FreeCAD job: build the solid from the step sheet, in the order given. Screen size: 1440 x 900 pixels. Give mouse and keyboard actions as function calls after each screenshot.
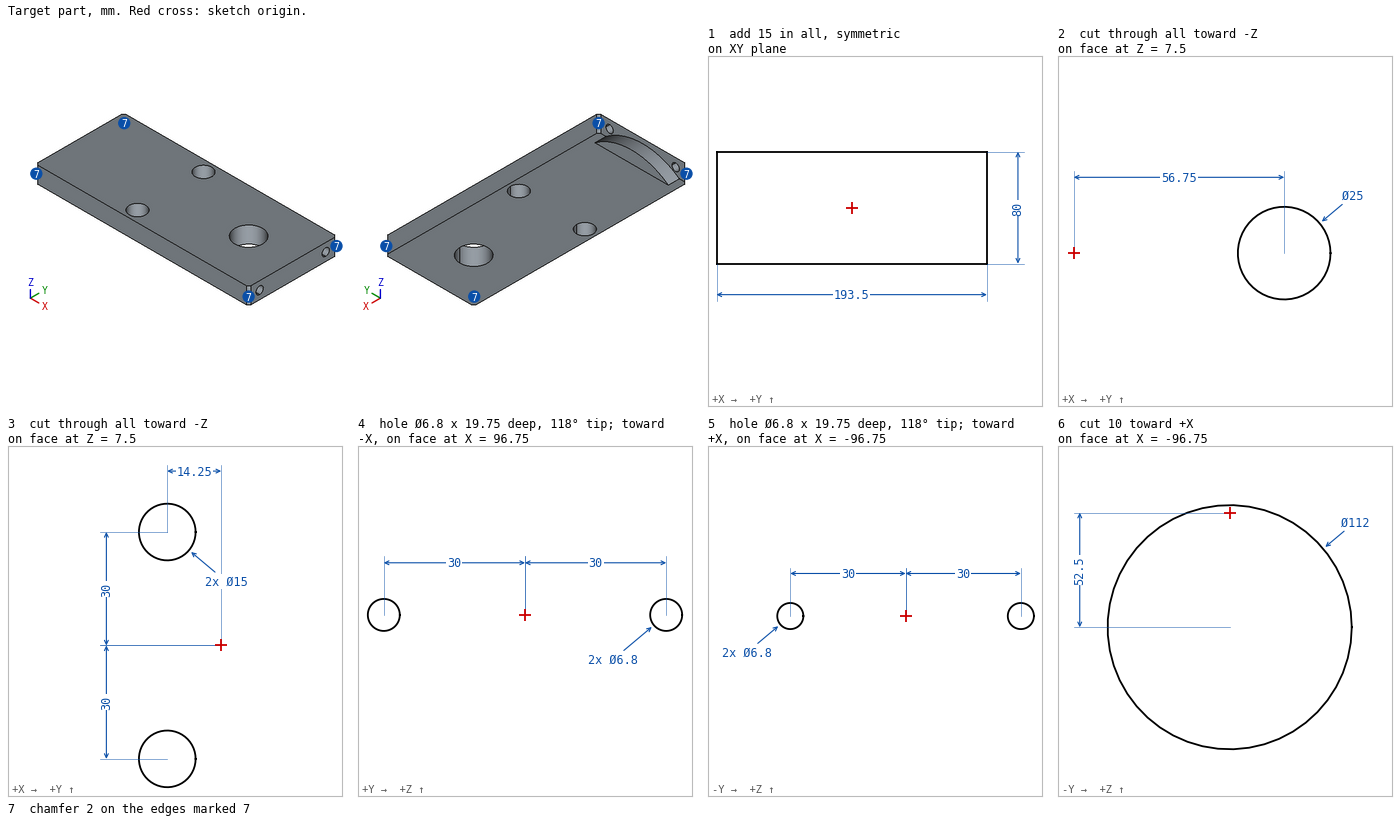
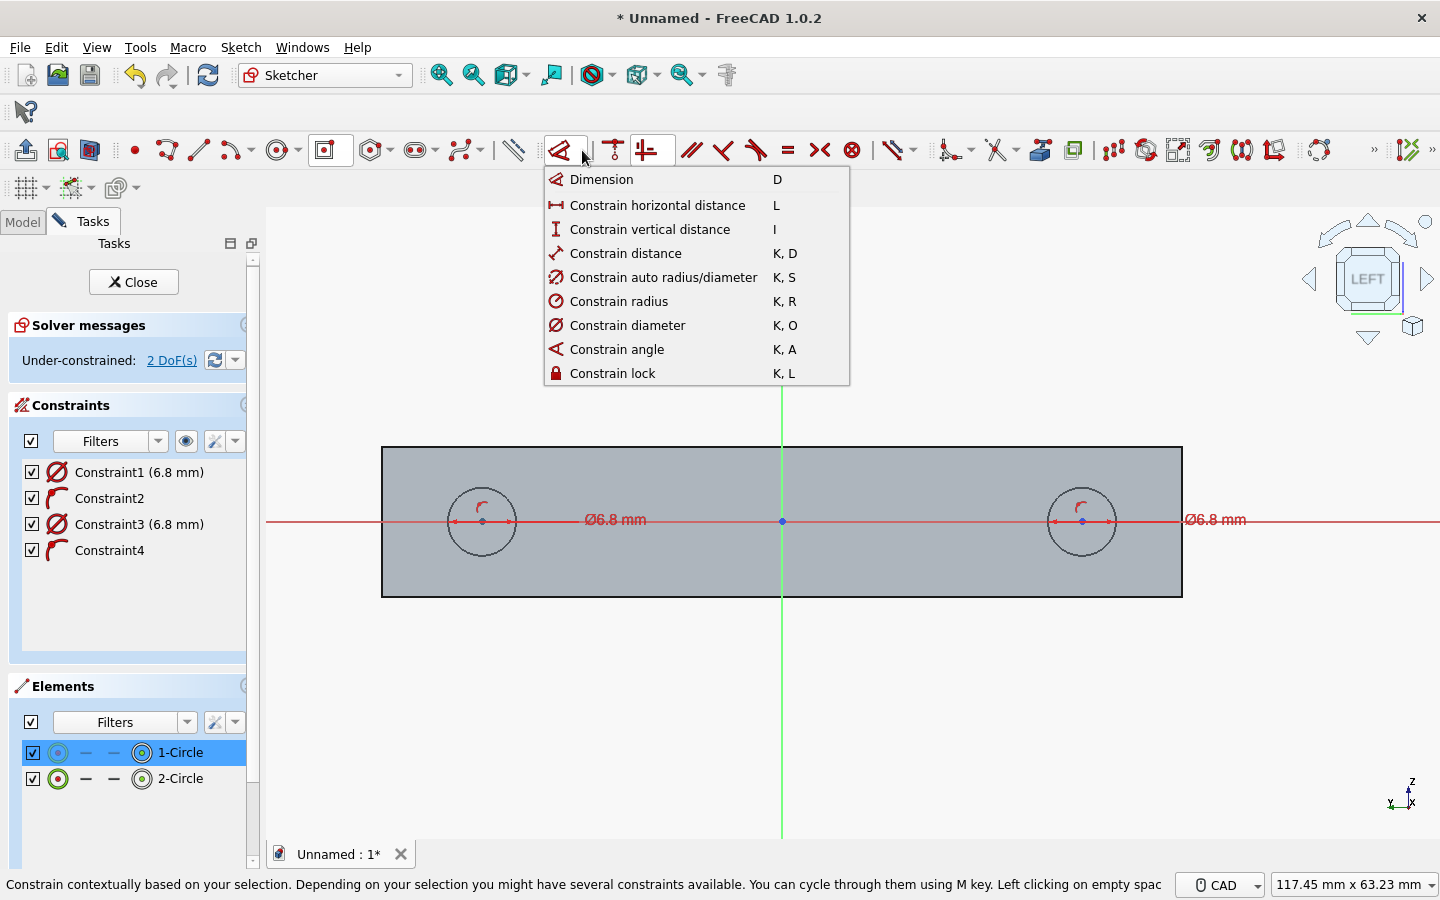
click(697, 205)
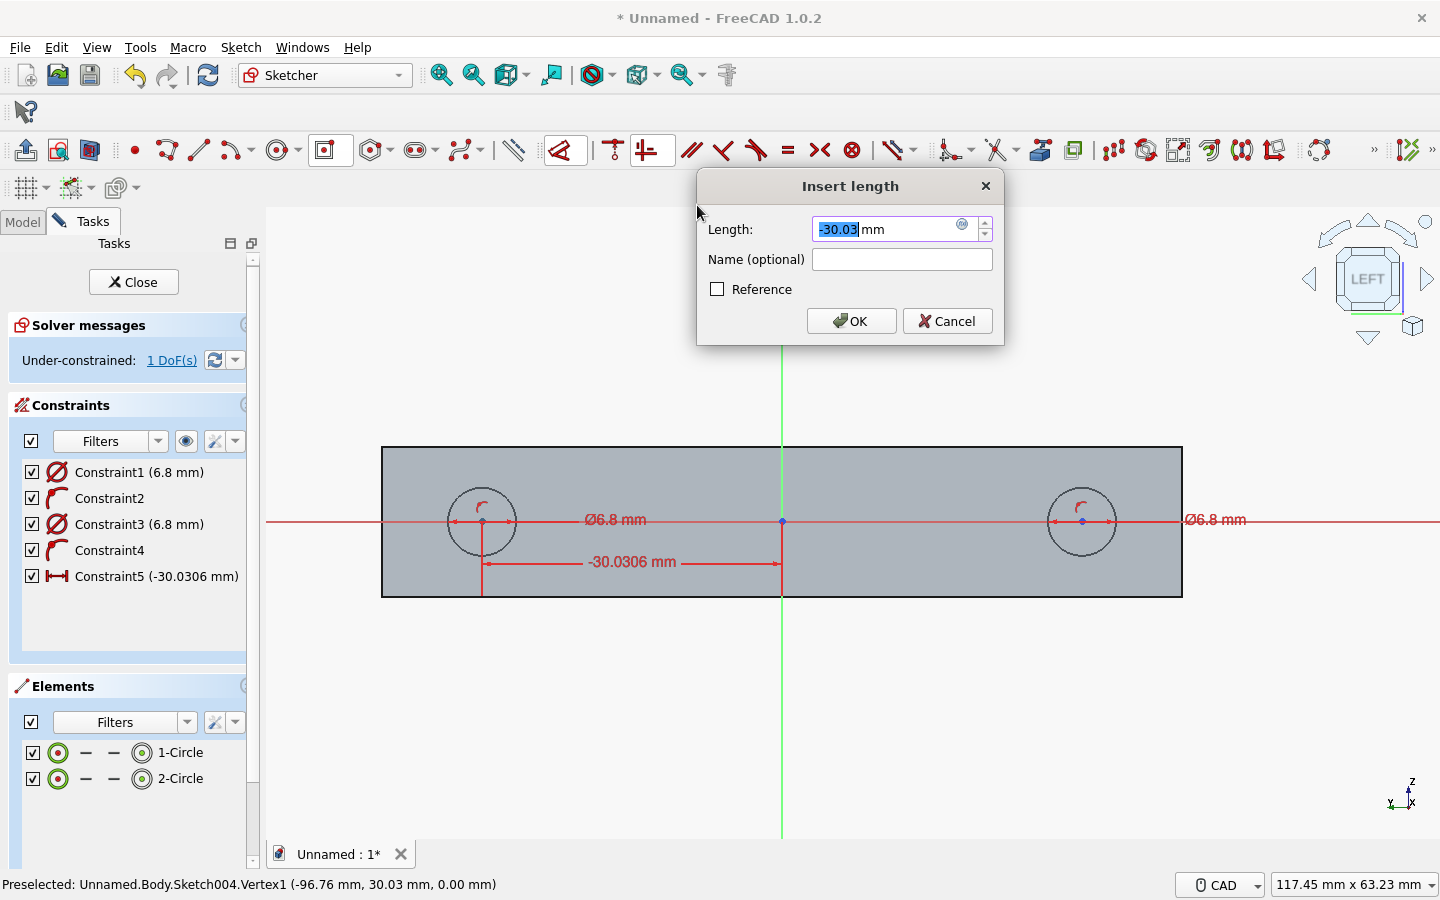
text(-30)
key(Return)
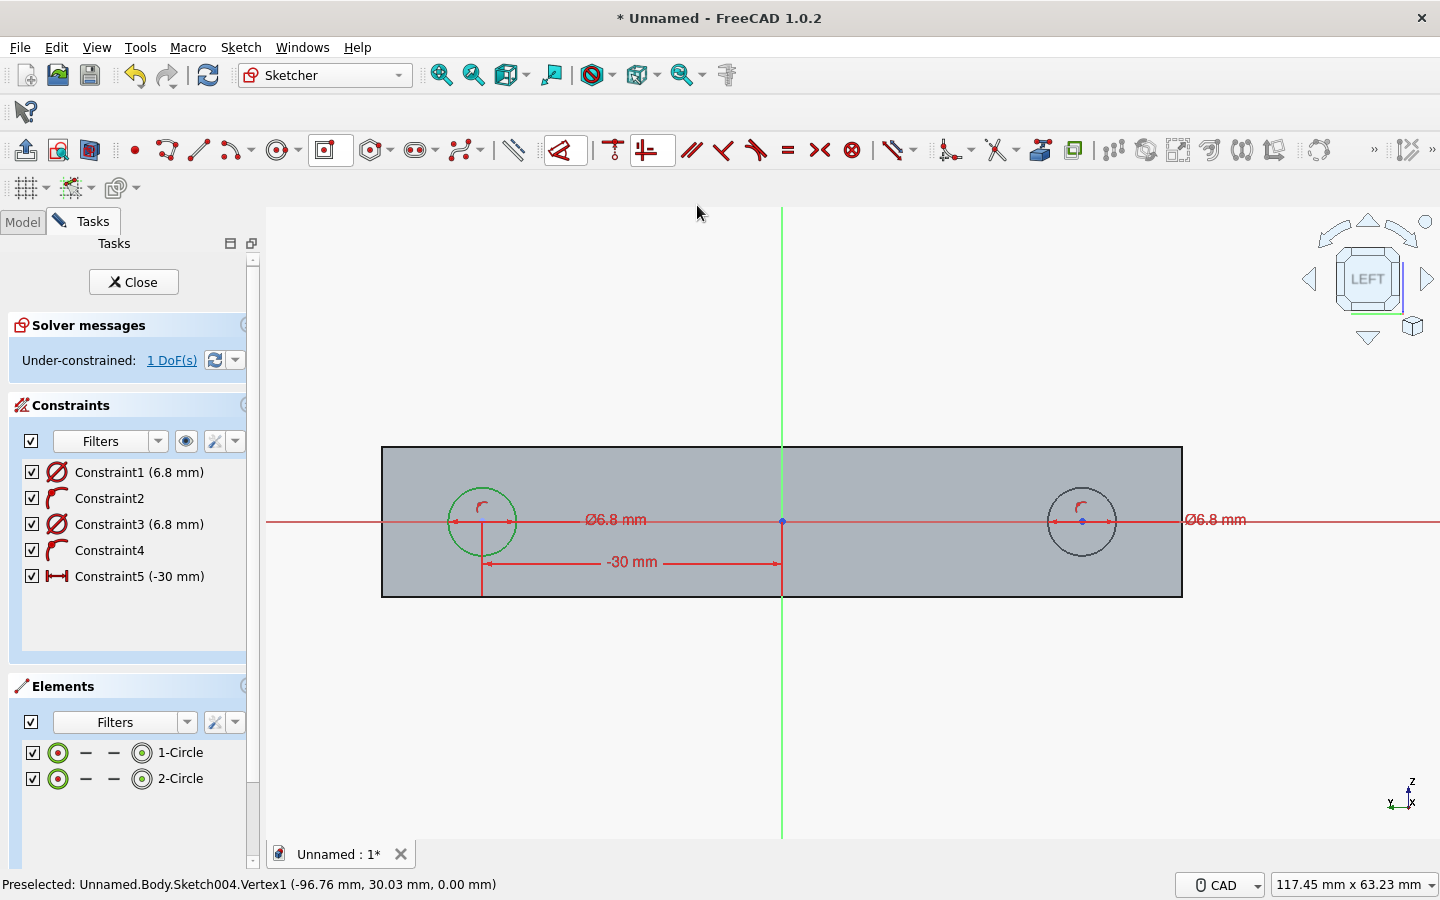
click(1082, 522)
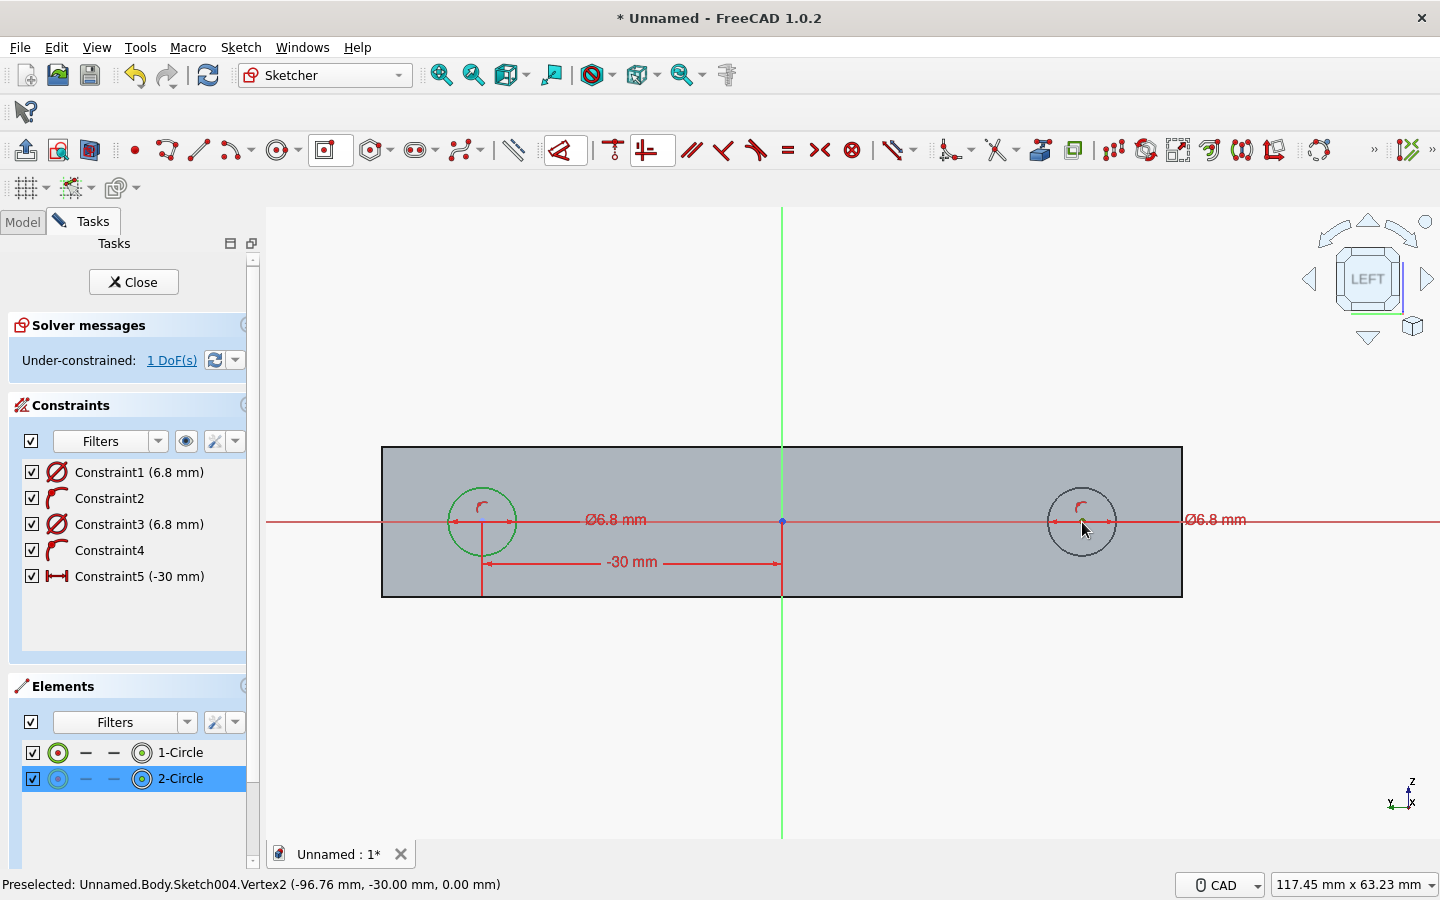
click(582, 150)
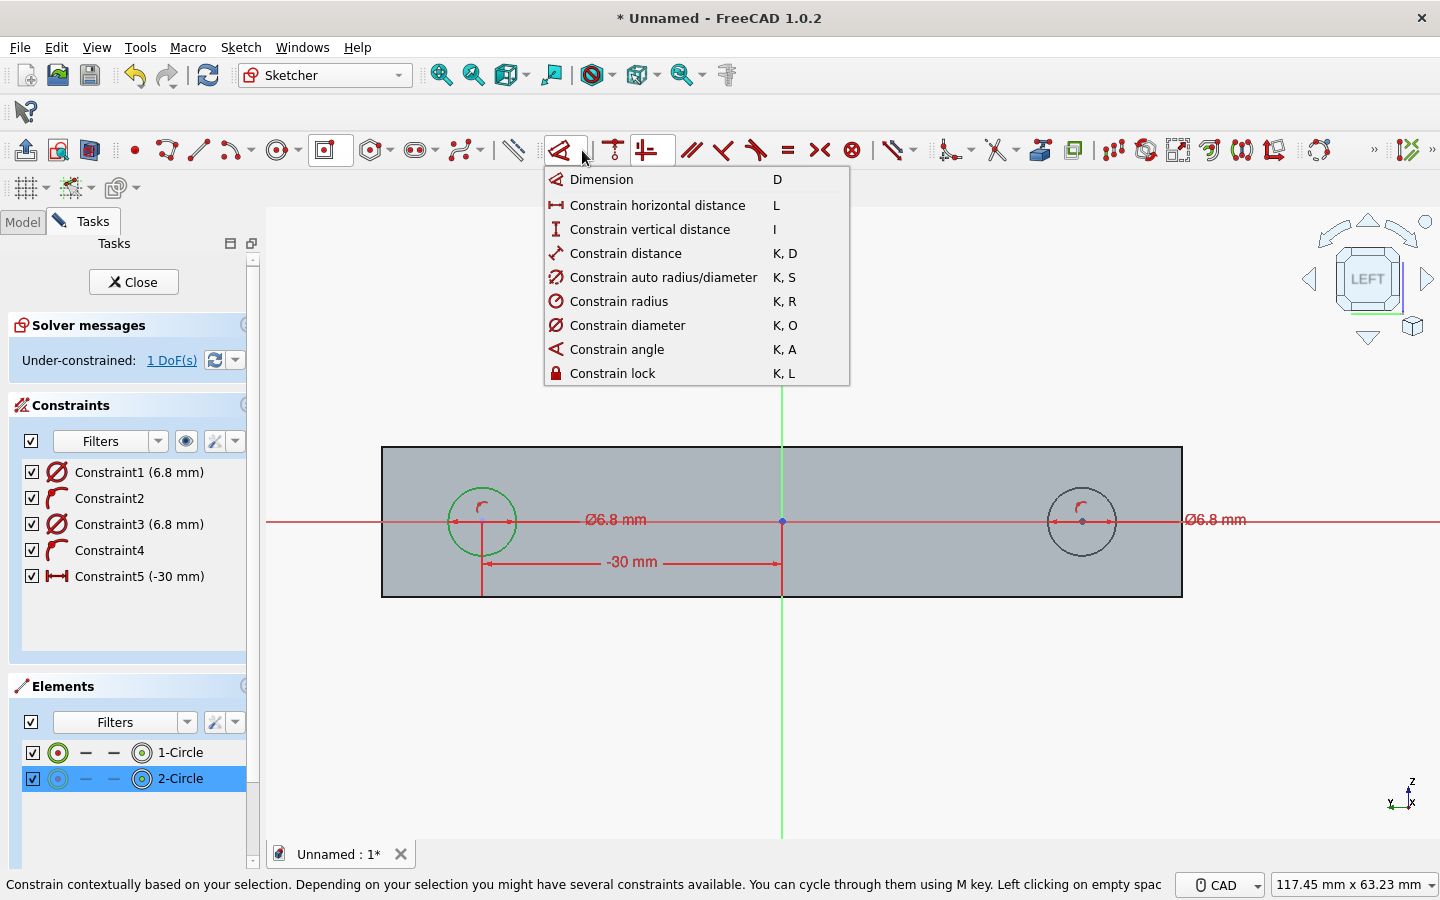
click(697, 205)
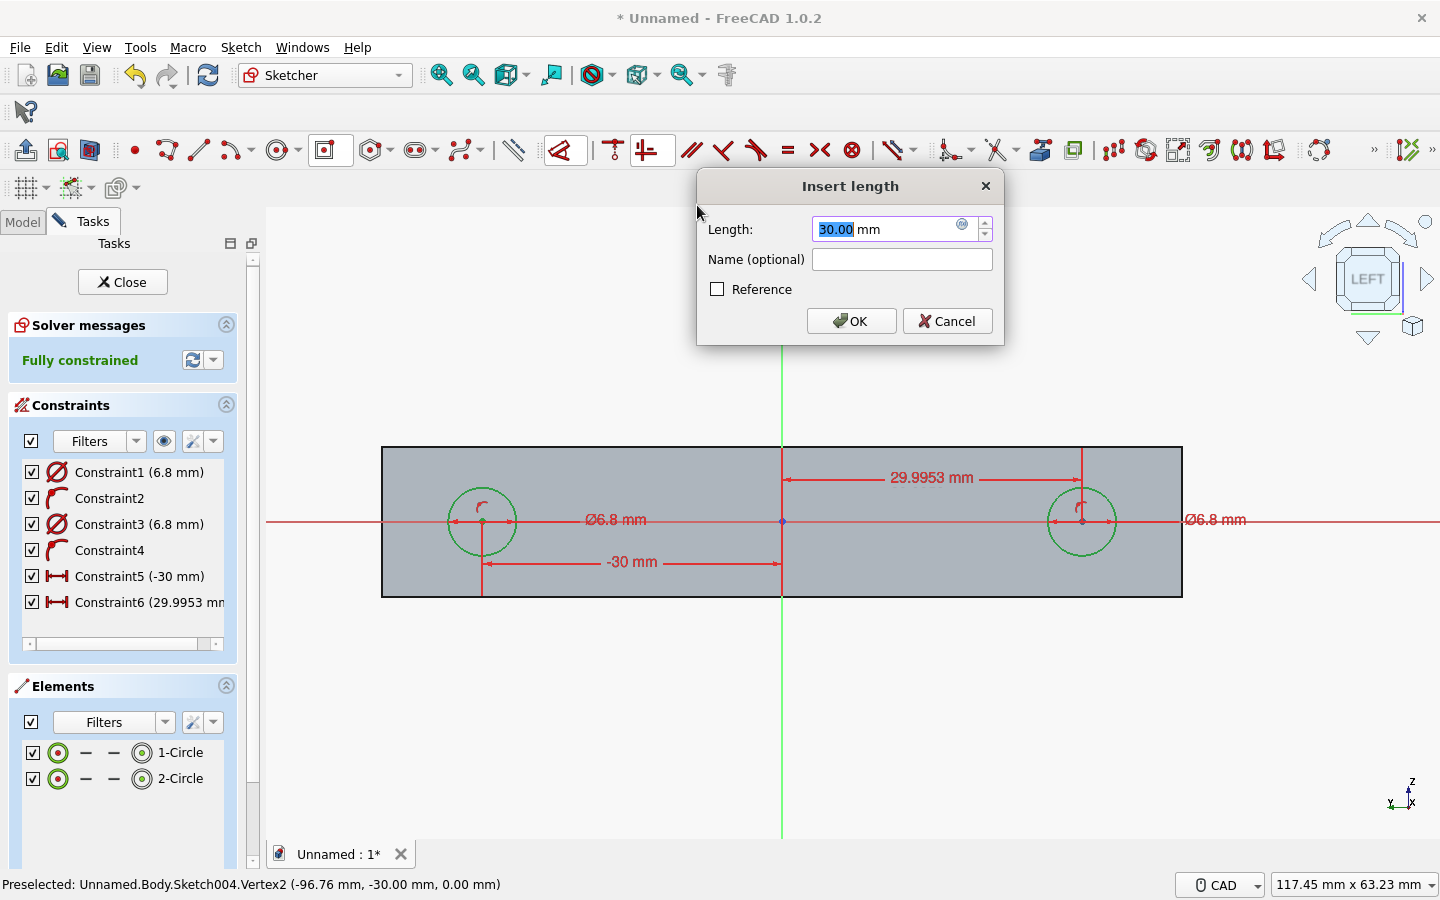
text(30)
key(Return)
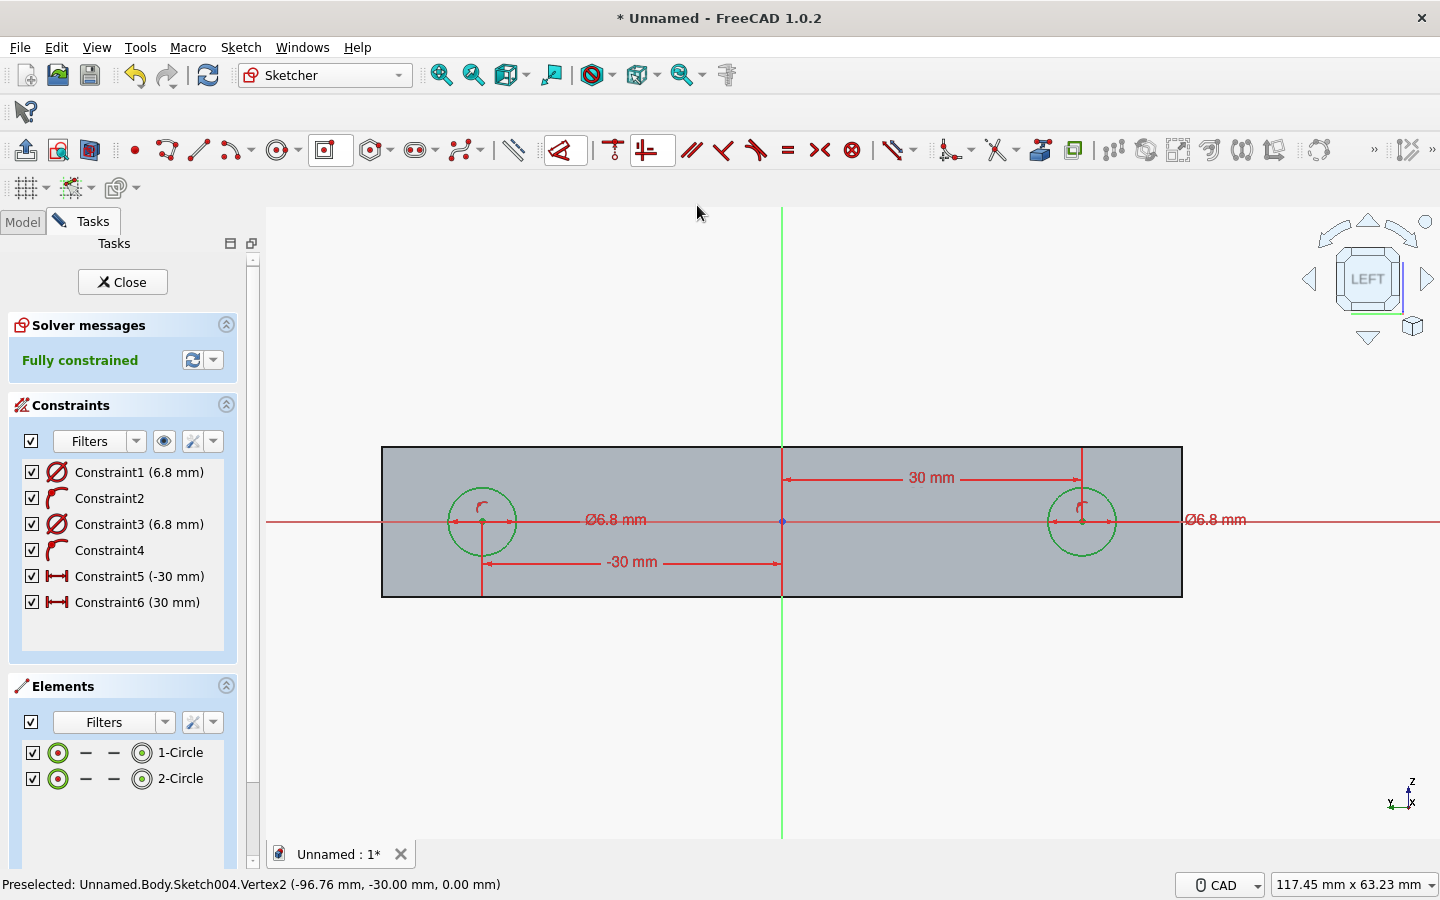
click(123, 282)